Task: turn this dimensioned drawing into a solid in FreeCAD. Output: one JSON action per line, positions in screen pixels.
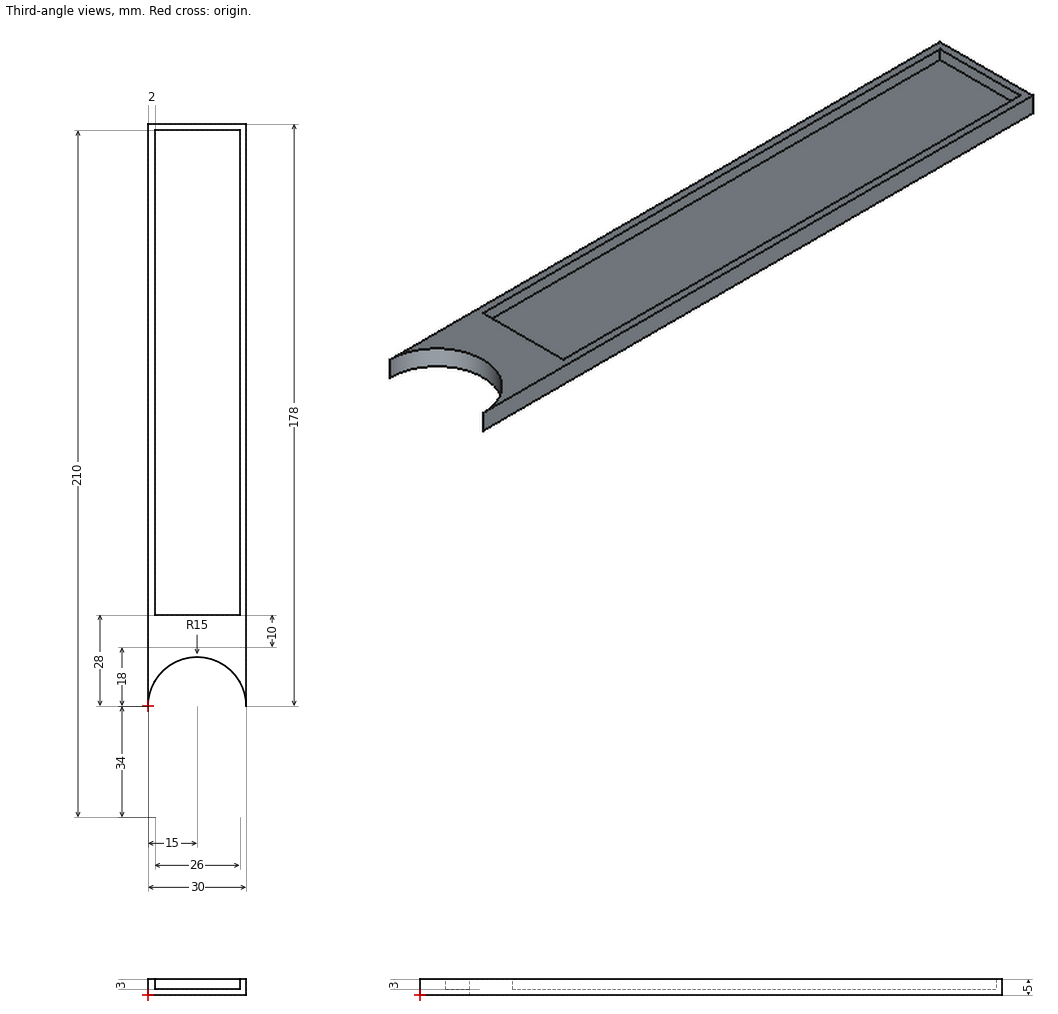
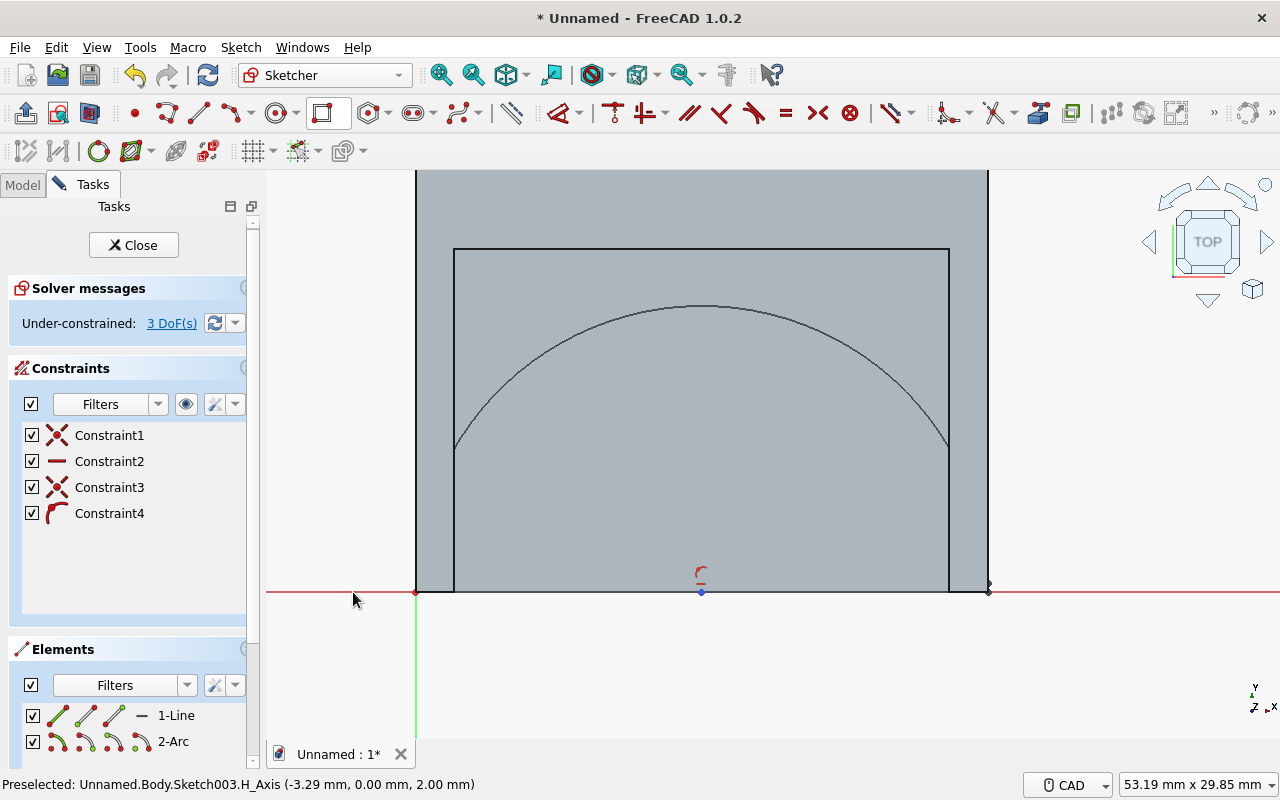
{"action": "left_click", "coordinate": [865, 357]}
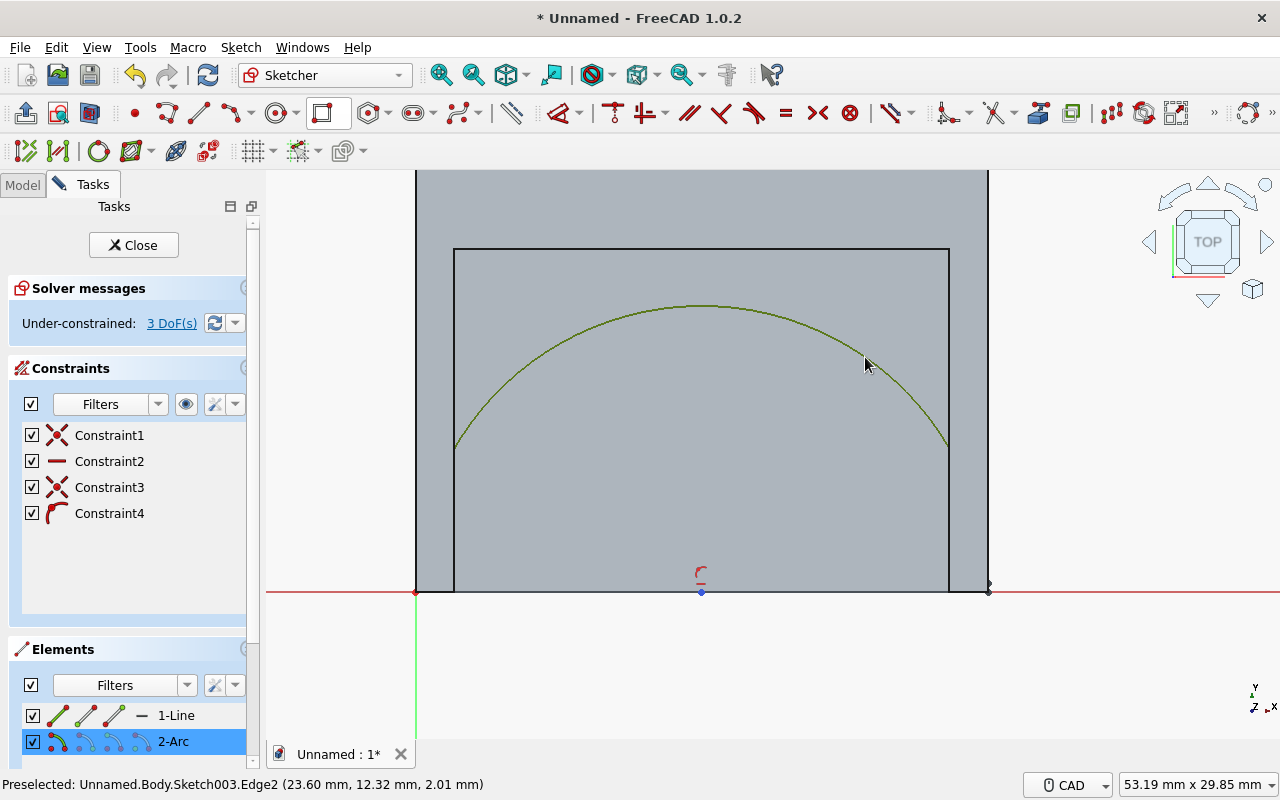
{"action": "key", "text": "k r"}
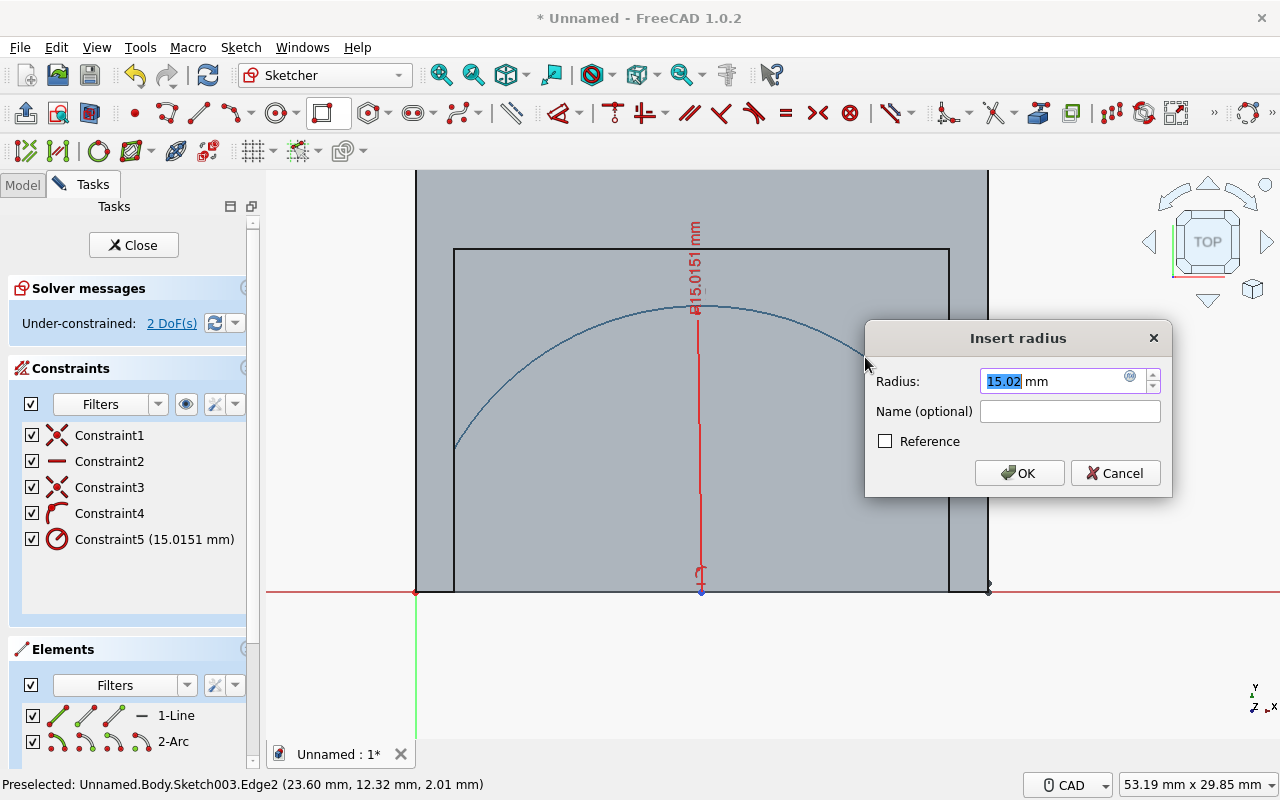
{"action": "type", "text": "15"}
{"action": "key", "text": "Return"}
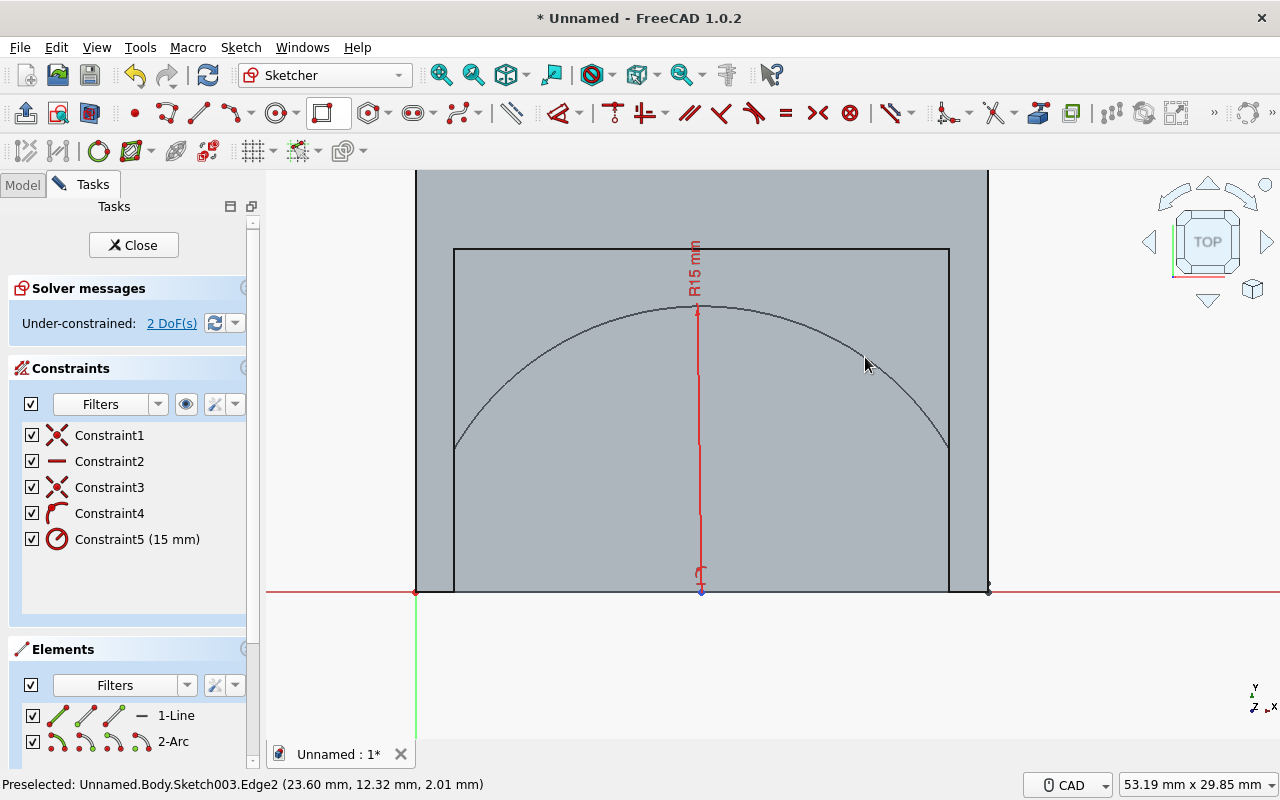
{"action": "left_click", "coordinate": [987, 584]}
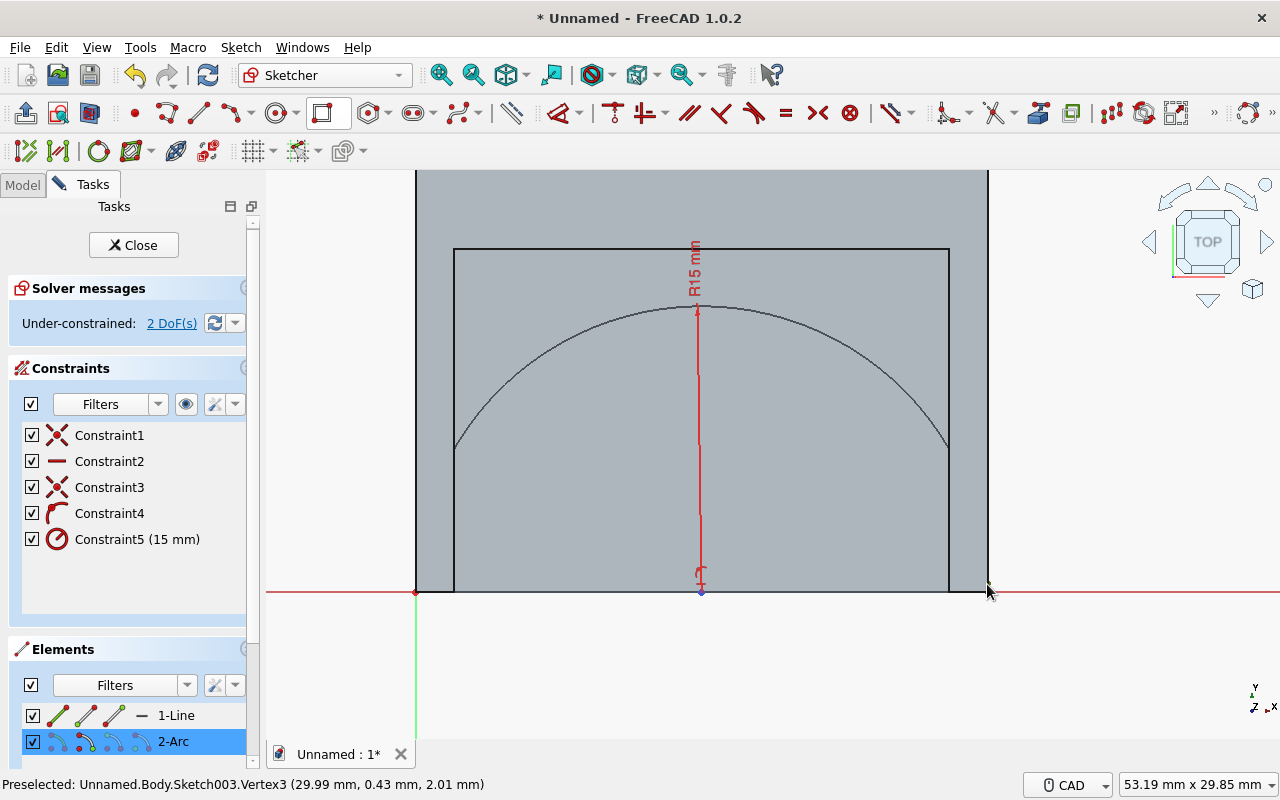
{"action": "left_click", "coordinate": [353, 592]}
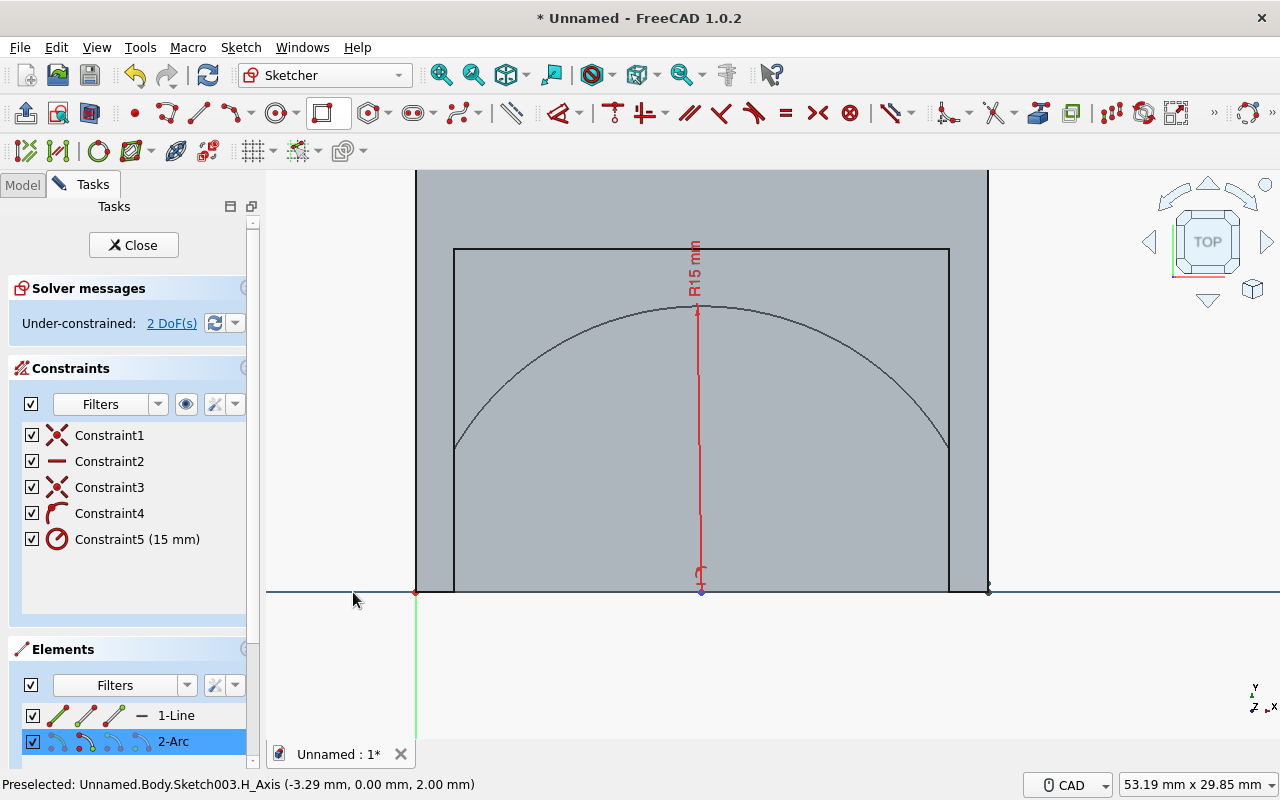
{"action": "left_click", "coordinate": [614, 114]}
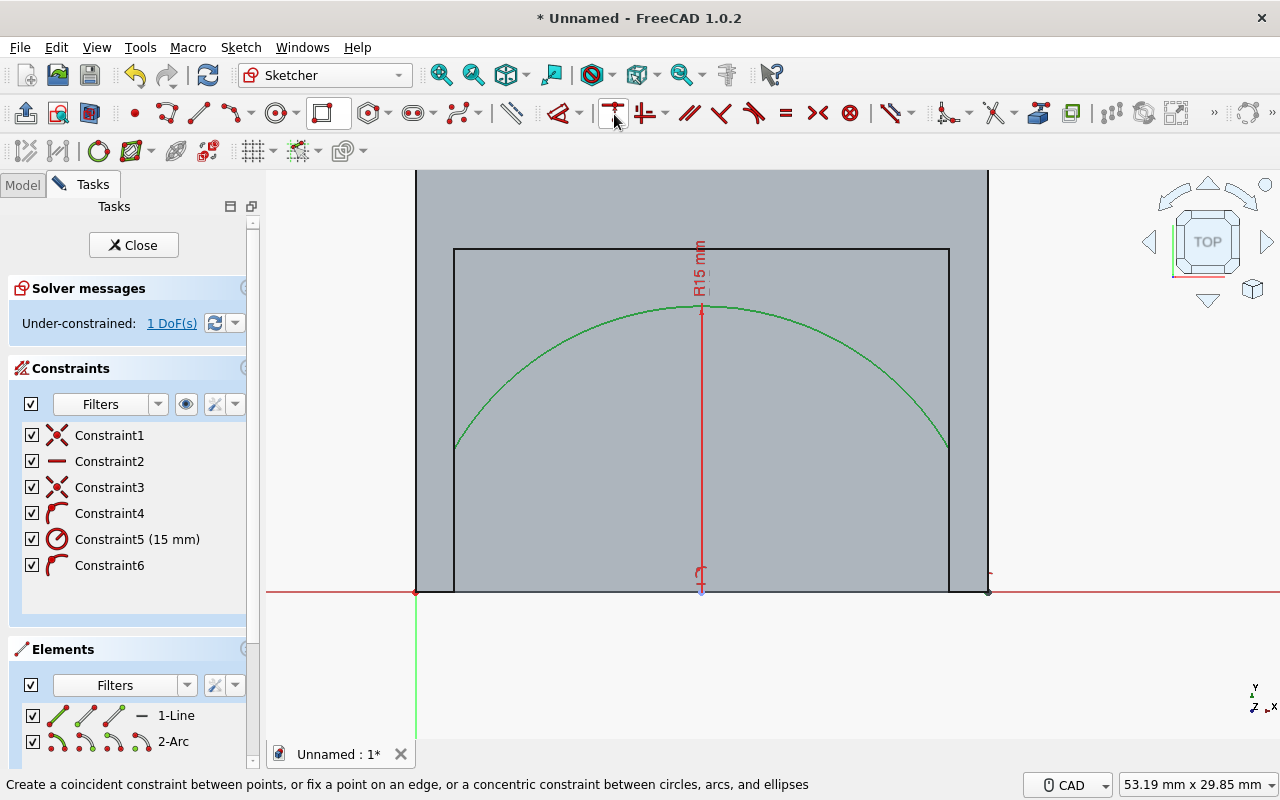
{"action": "left_click", "coordinate": [587, 592]}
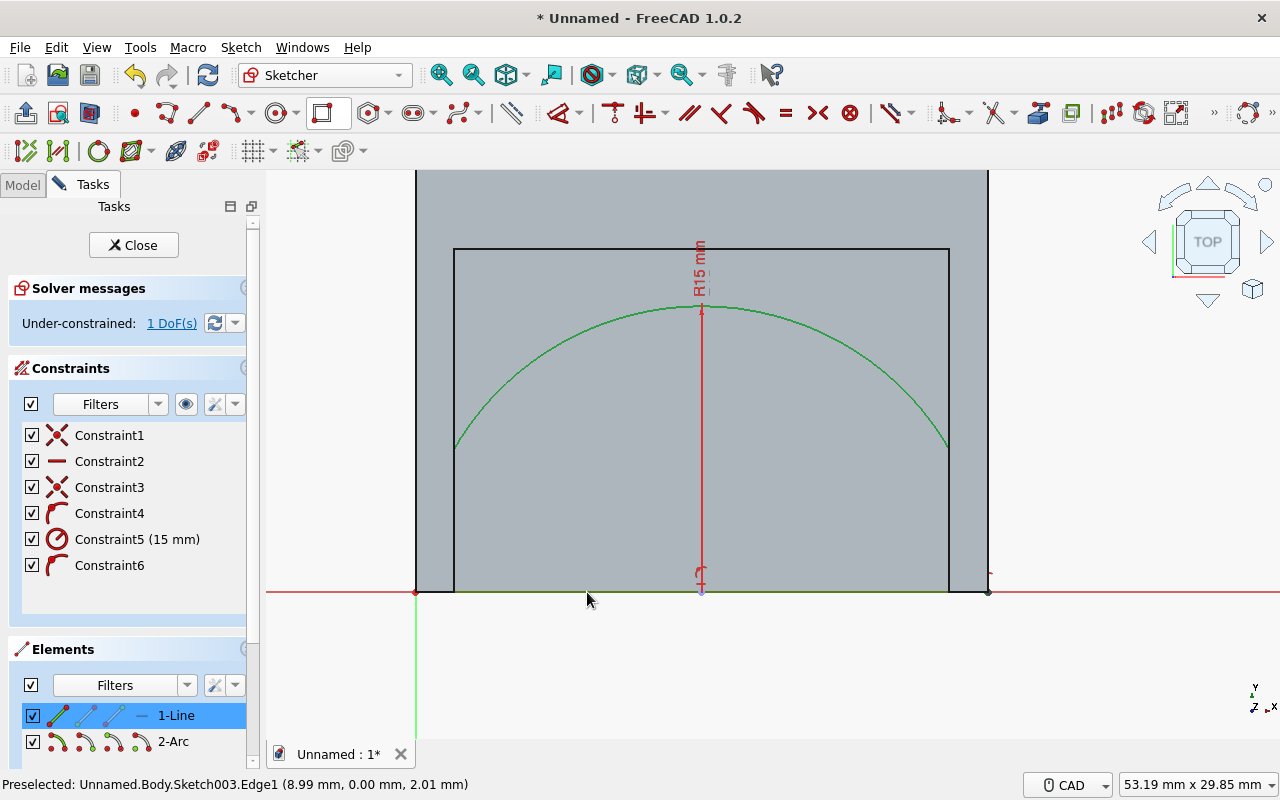
{"action": "key", "text": "l"}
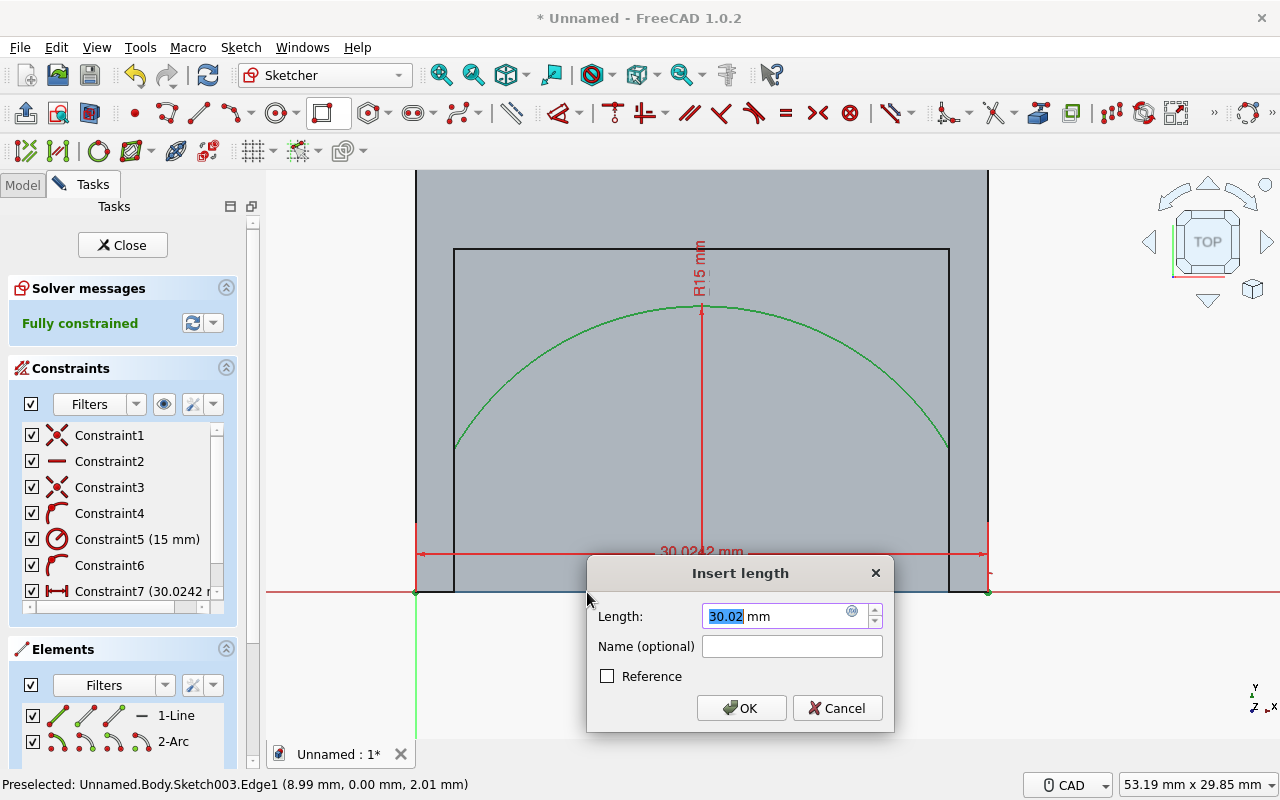
{"action": "type", "text": "30"}
{"action": "key", "text": "Return"}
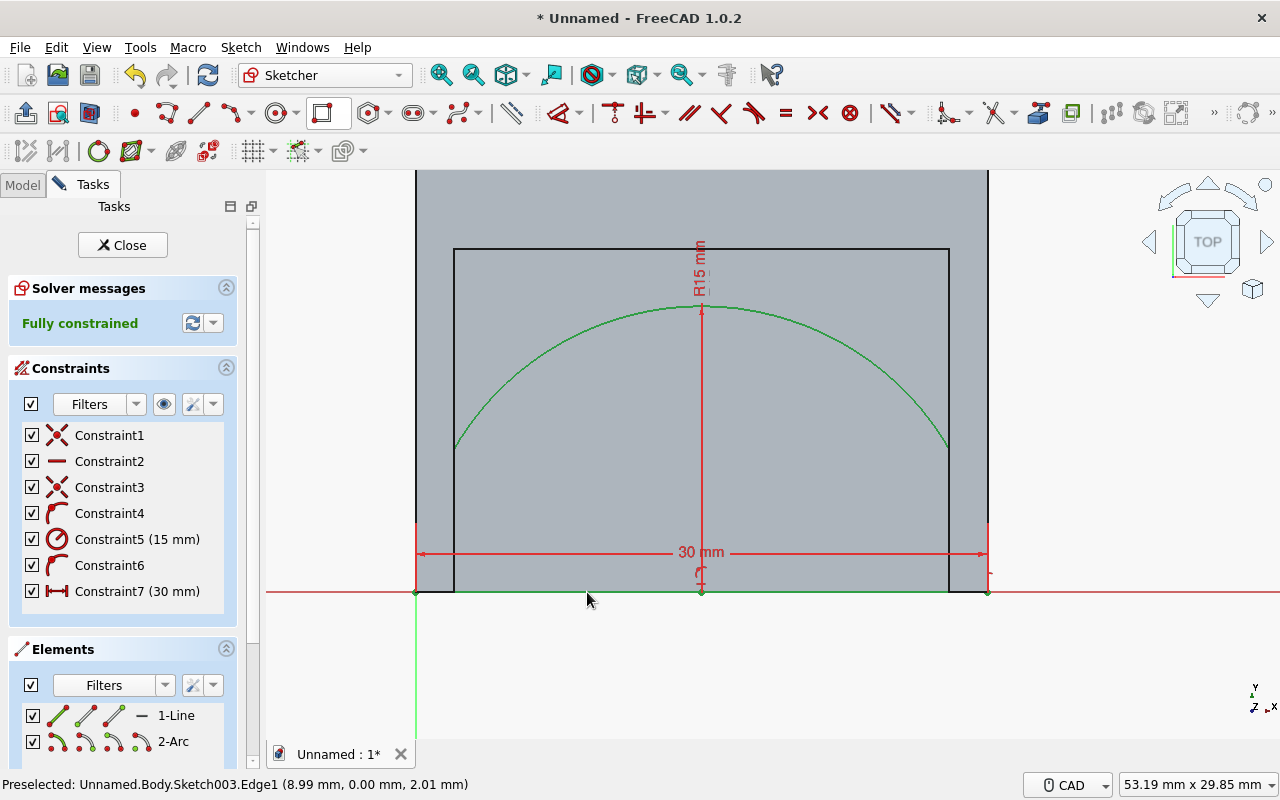
{"action": "left_click", "coordinate": [123, 245]}